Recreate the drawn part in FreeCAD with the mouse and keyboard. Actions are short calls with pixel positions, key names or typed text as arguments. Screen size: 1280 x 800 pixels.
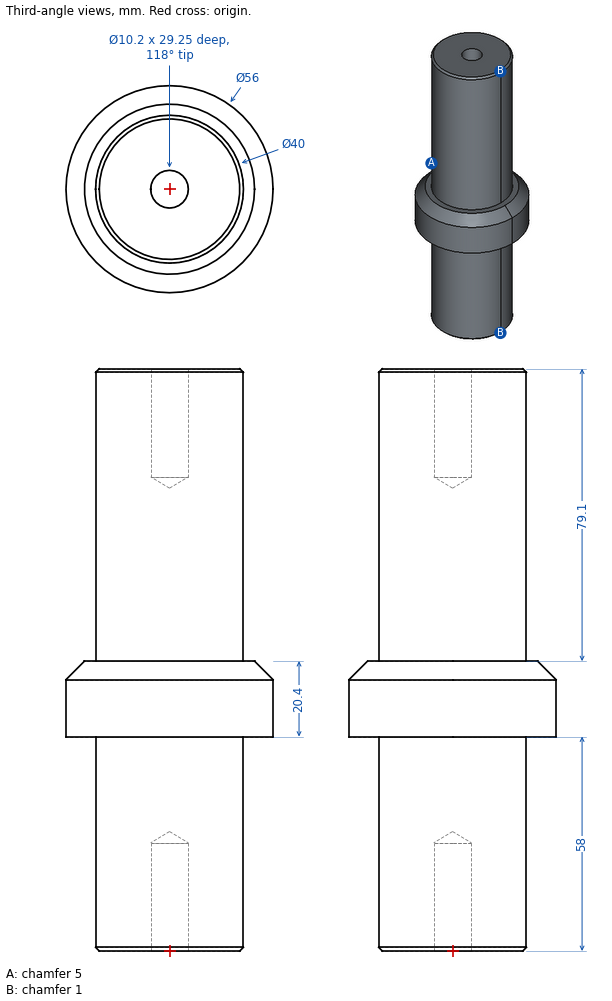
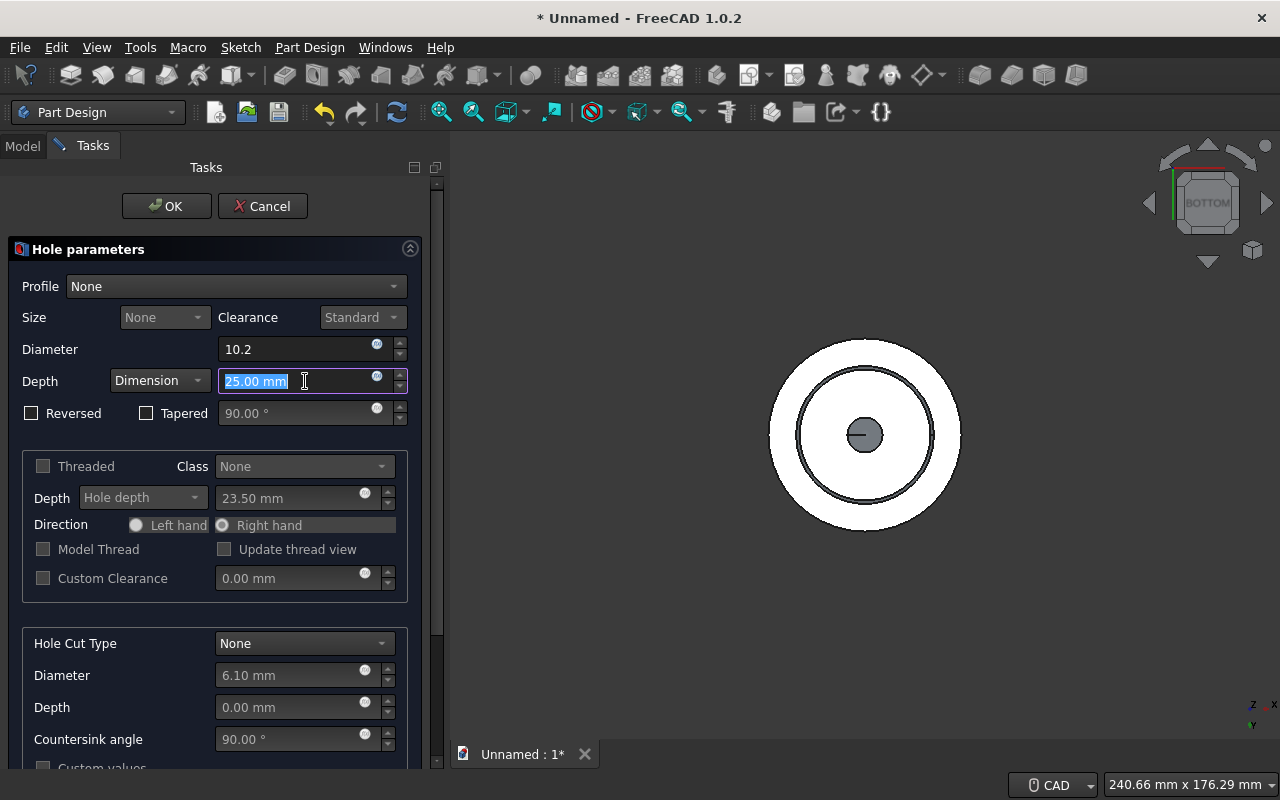
text(29.25)
key(Tab)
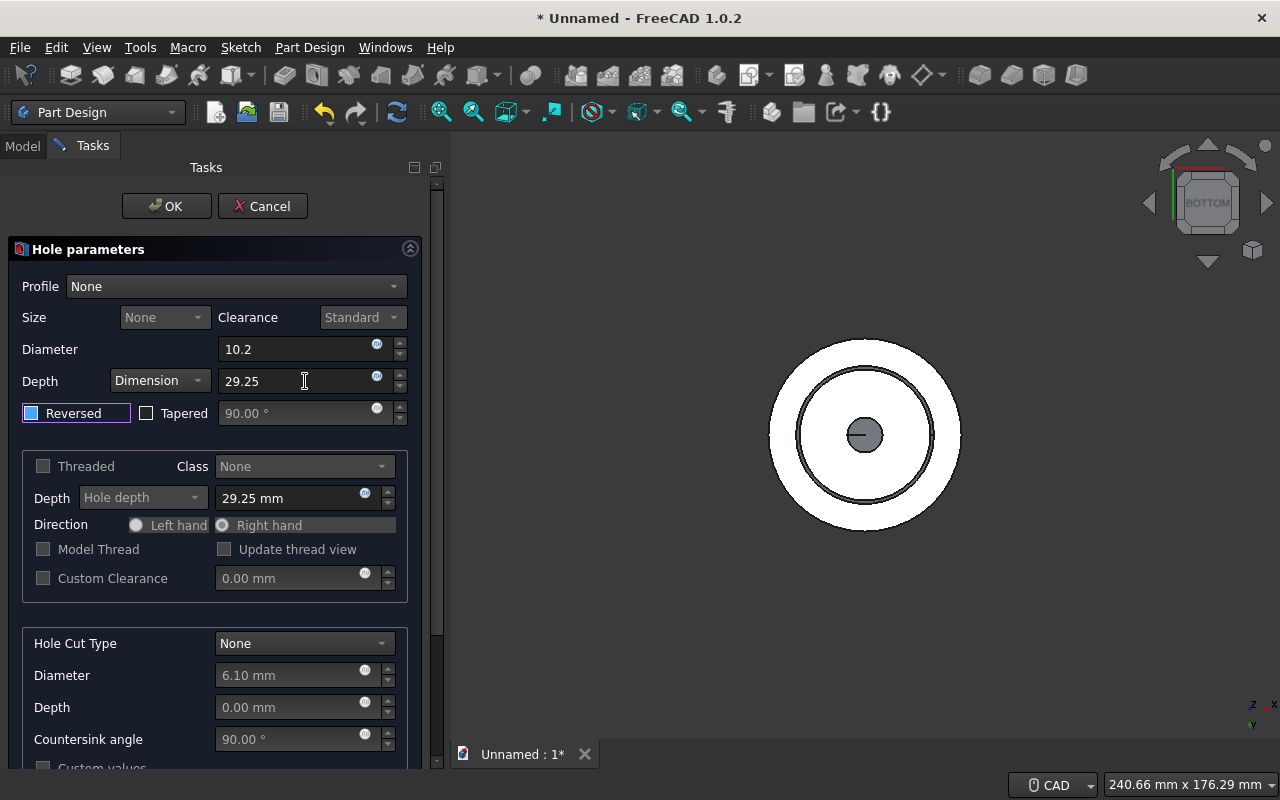
click(167, 206)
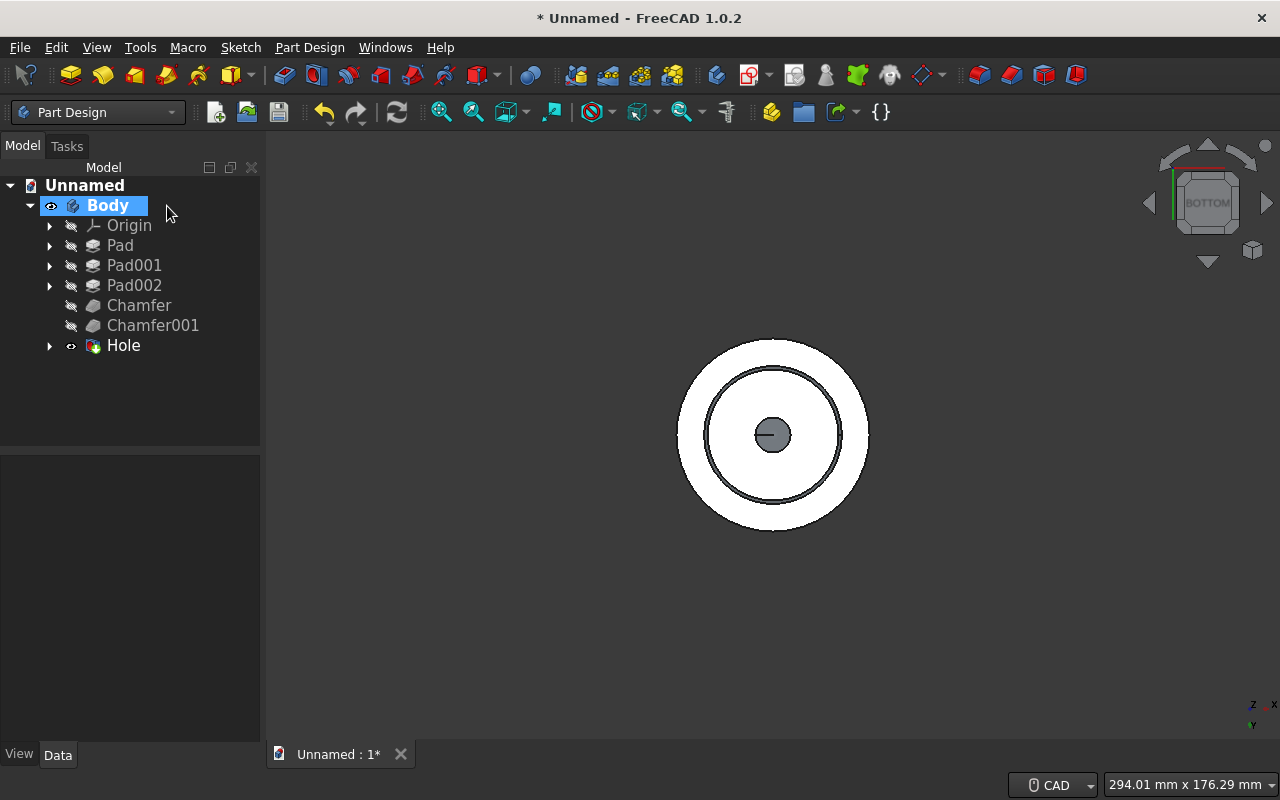
click(442, 112)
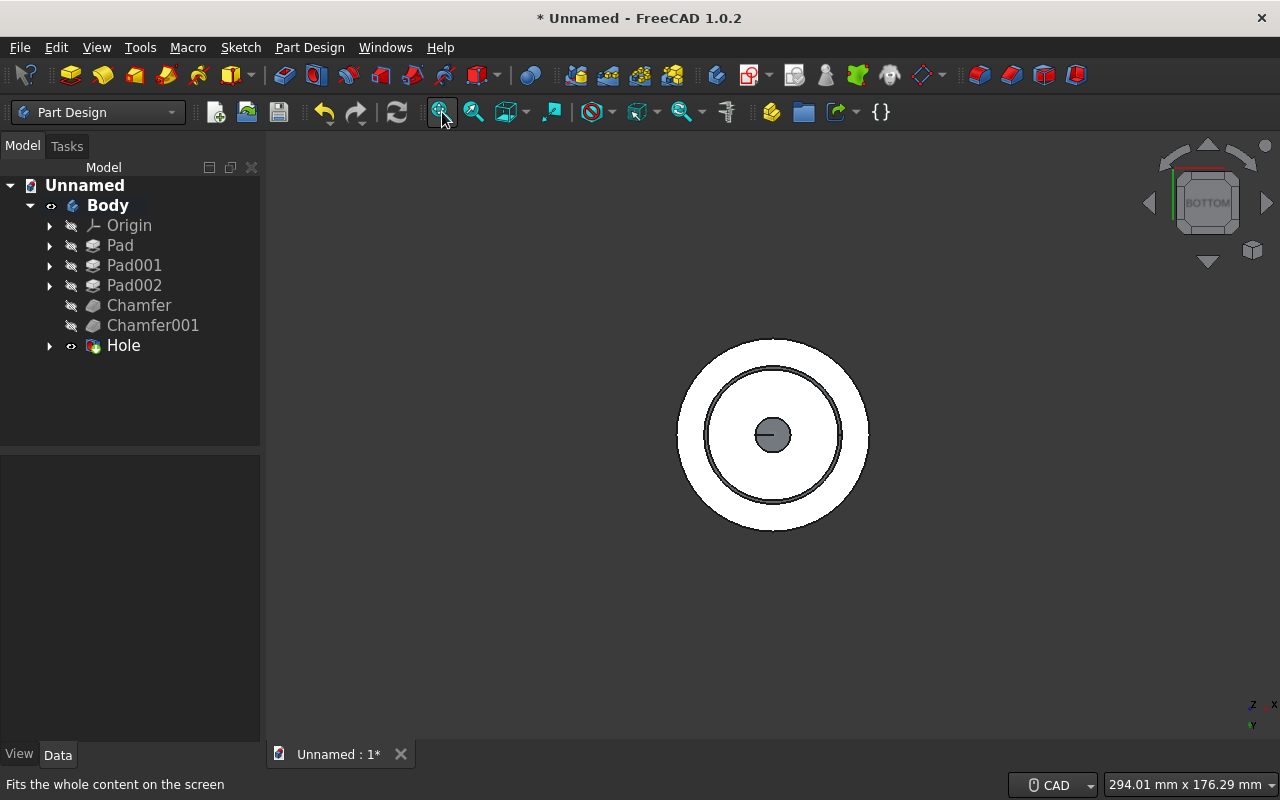
key(0)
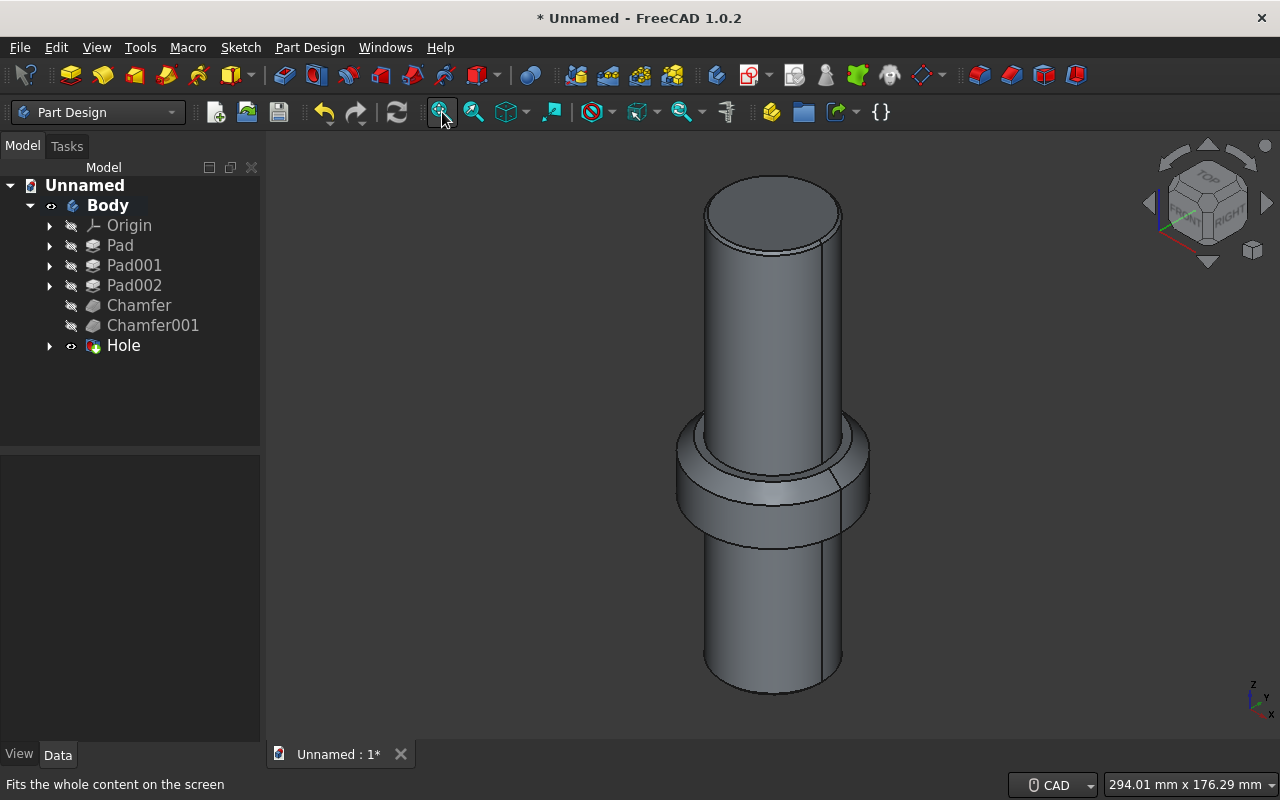
click(773, 212)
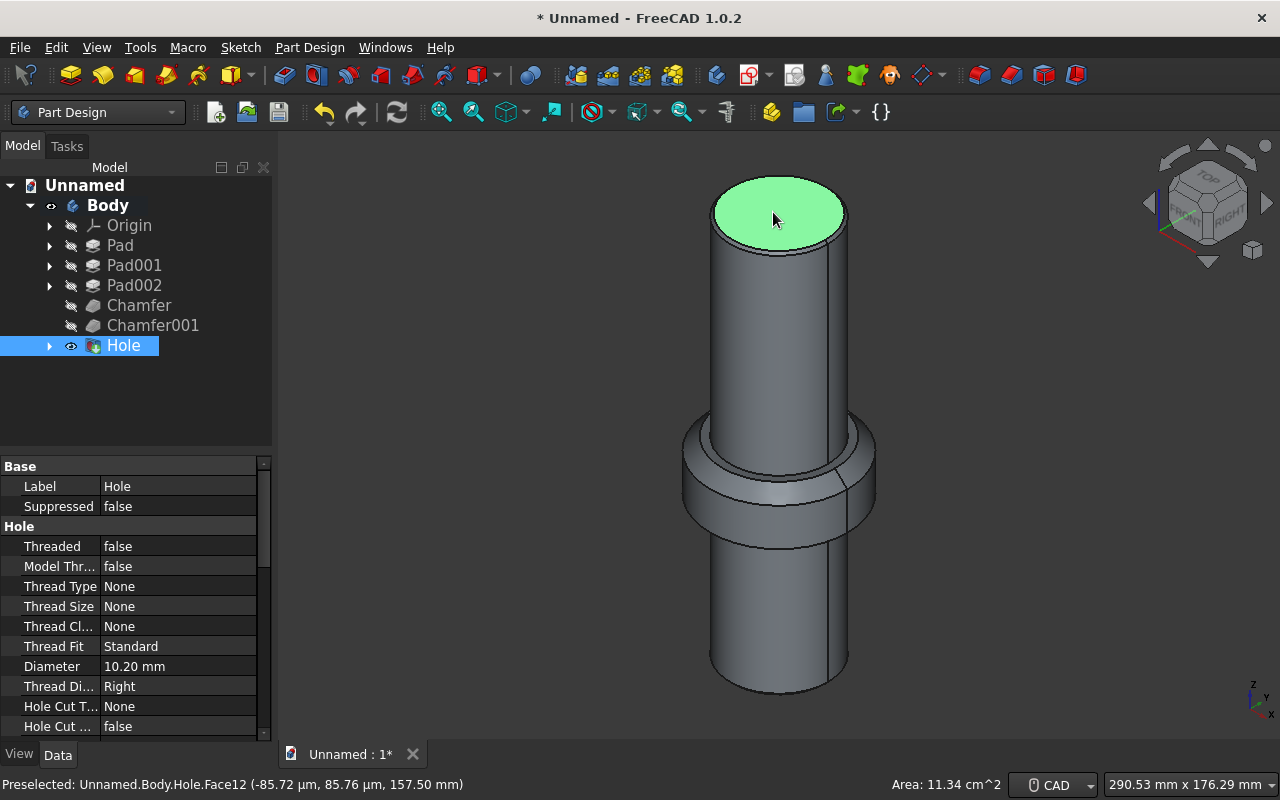
click(750, 76)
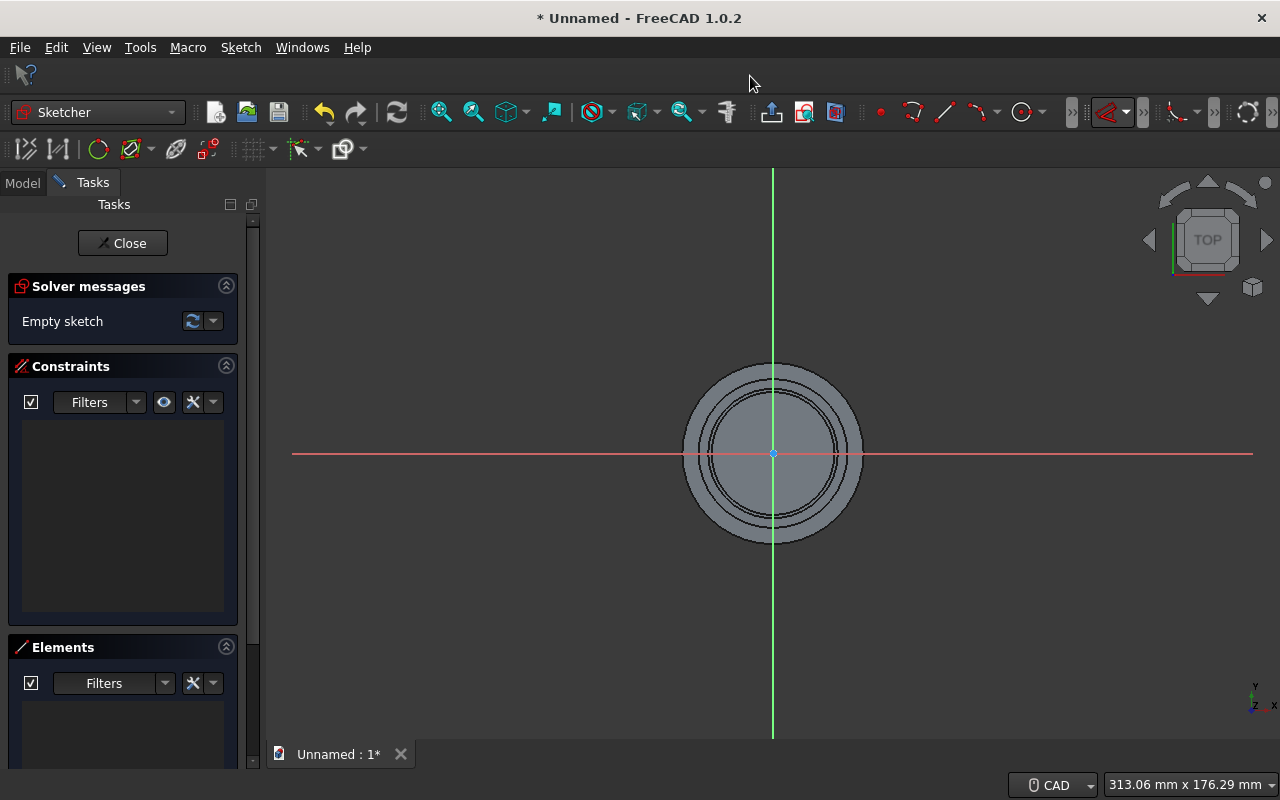
scroll(780, 454, up, 12)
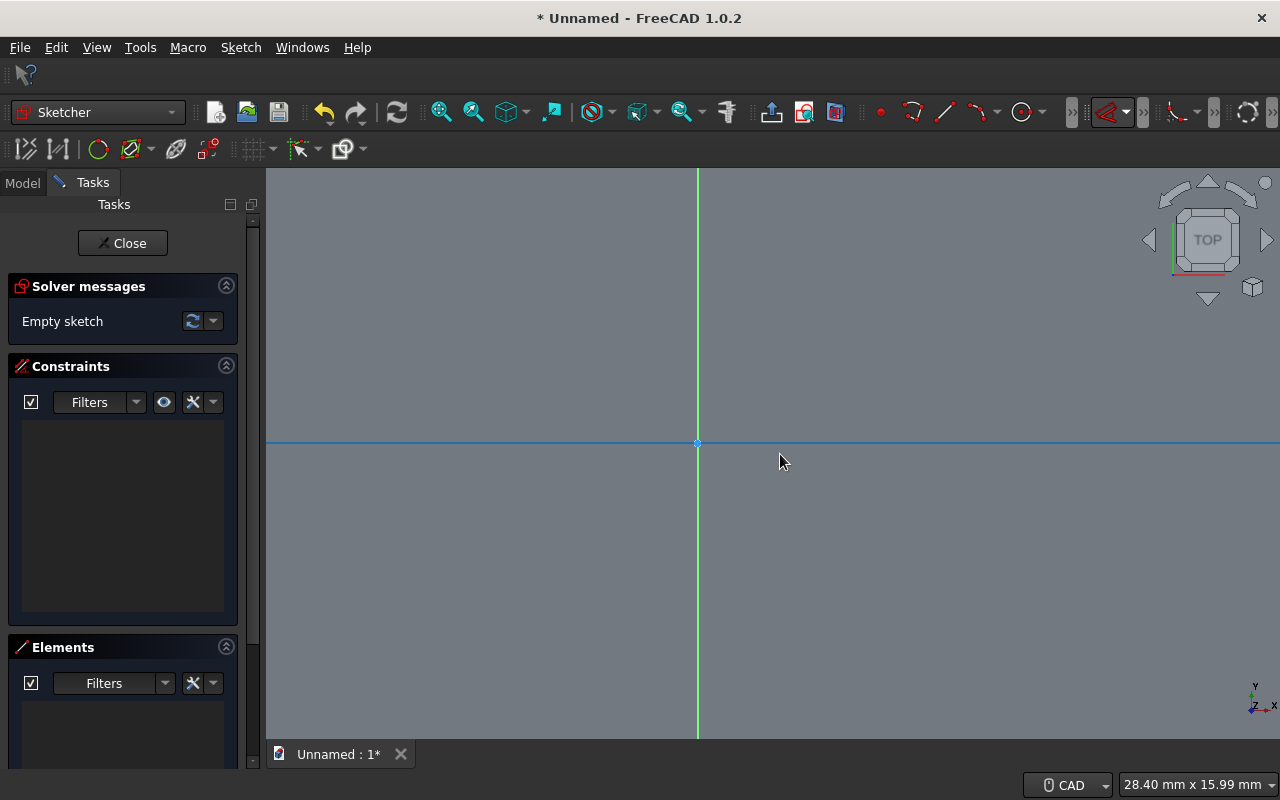
click(1022, 112)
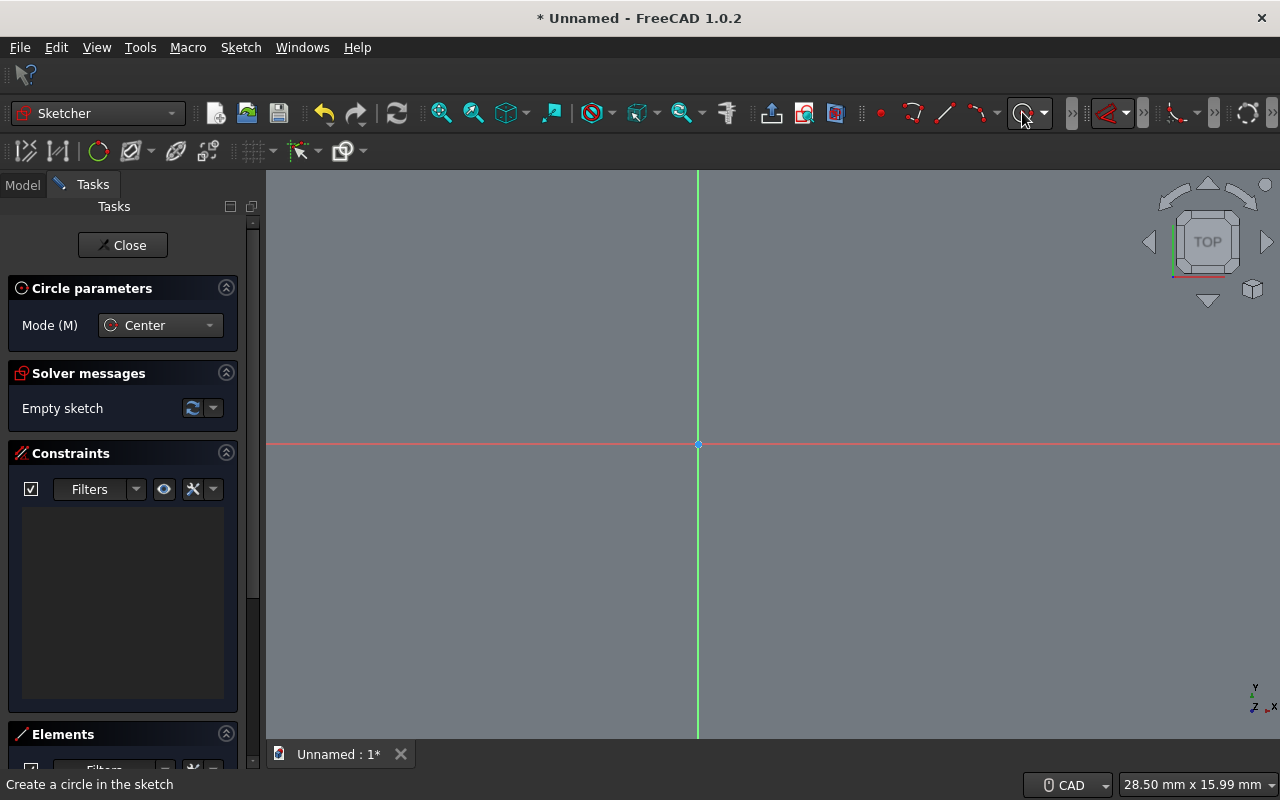
click(698, 444)
move(826, 316)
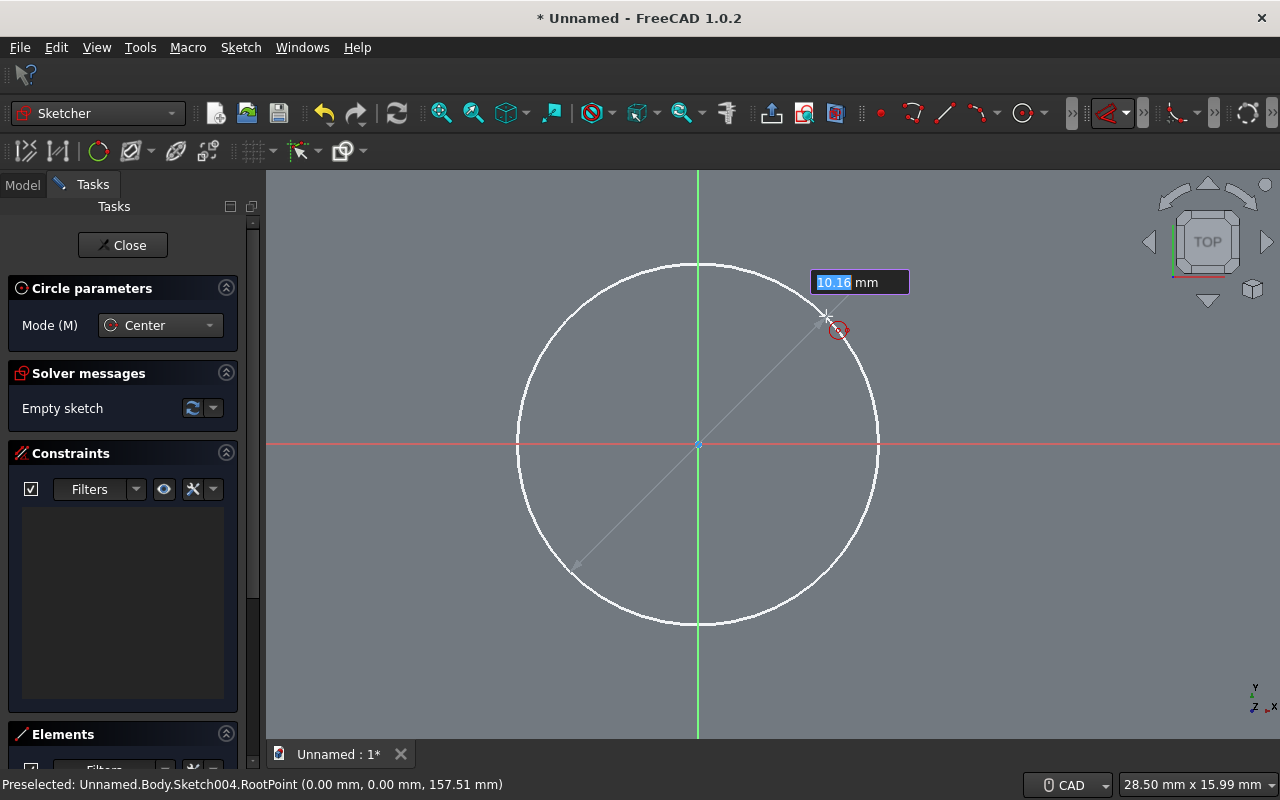
text(10.2)
key(Return)
key(Escape)